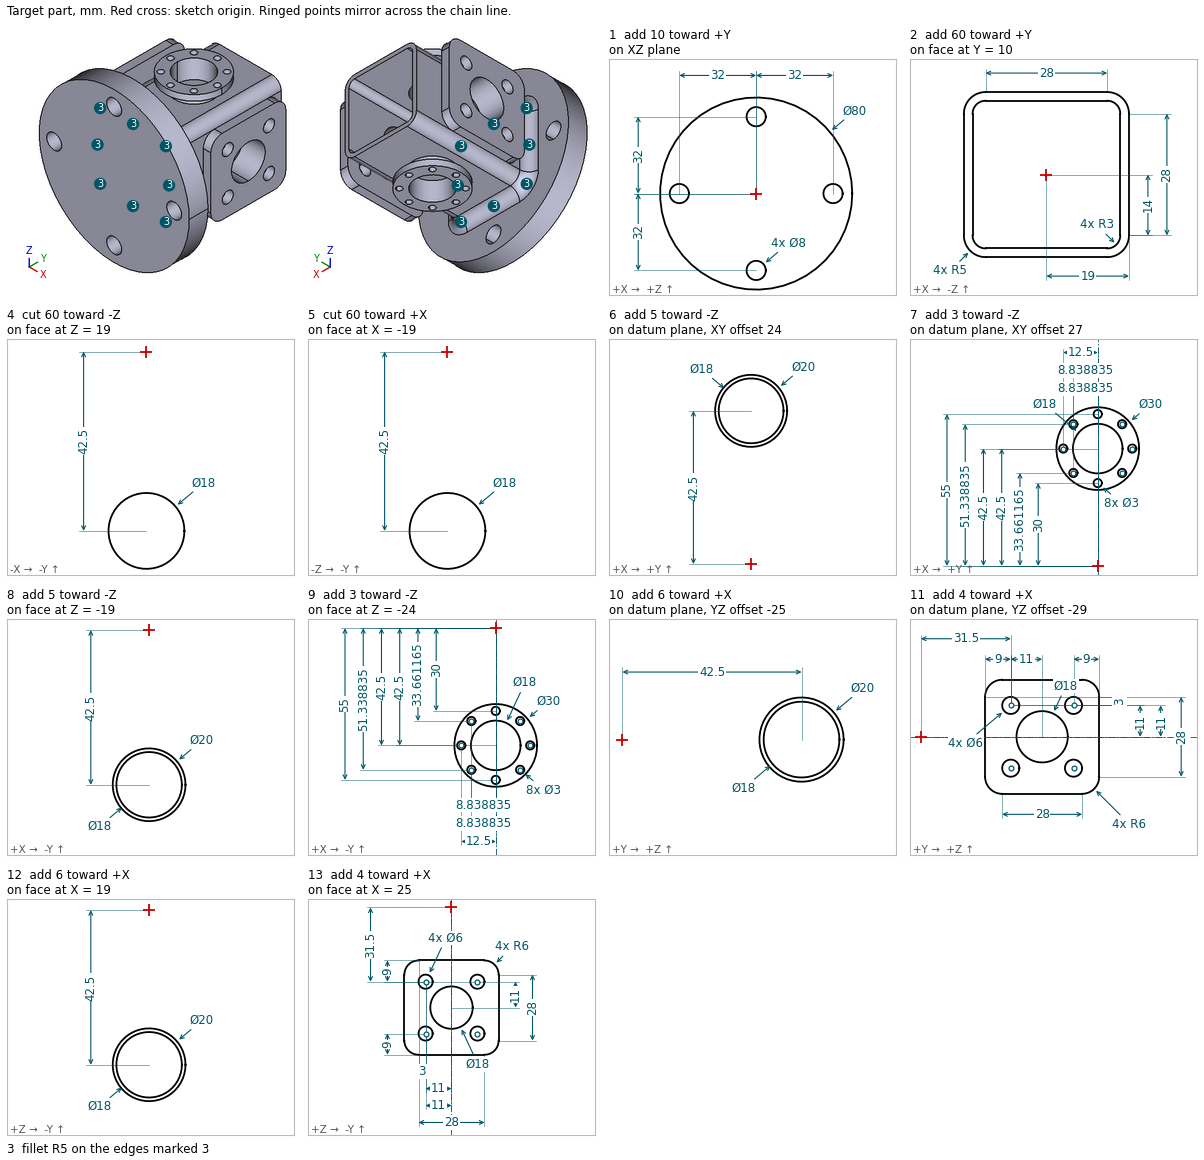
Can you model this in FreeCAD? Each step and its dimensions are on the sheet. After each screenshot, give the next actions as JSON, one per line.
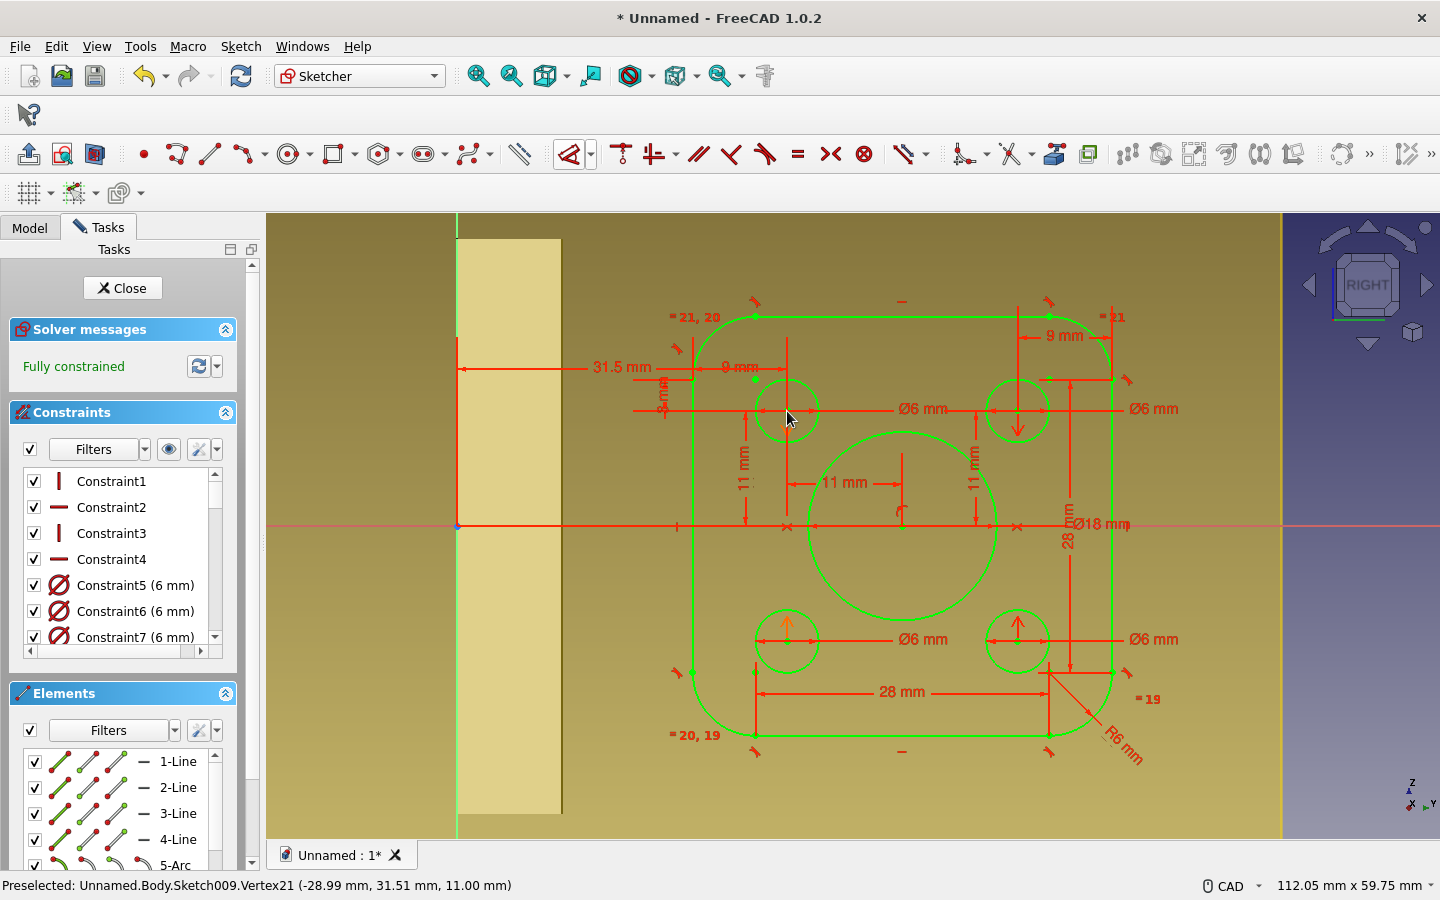
{"action": "left_click", "coordinate": [123, 288]}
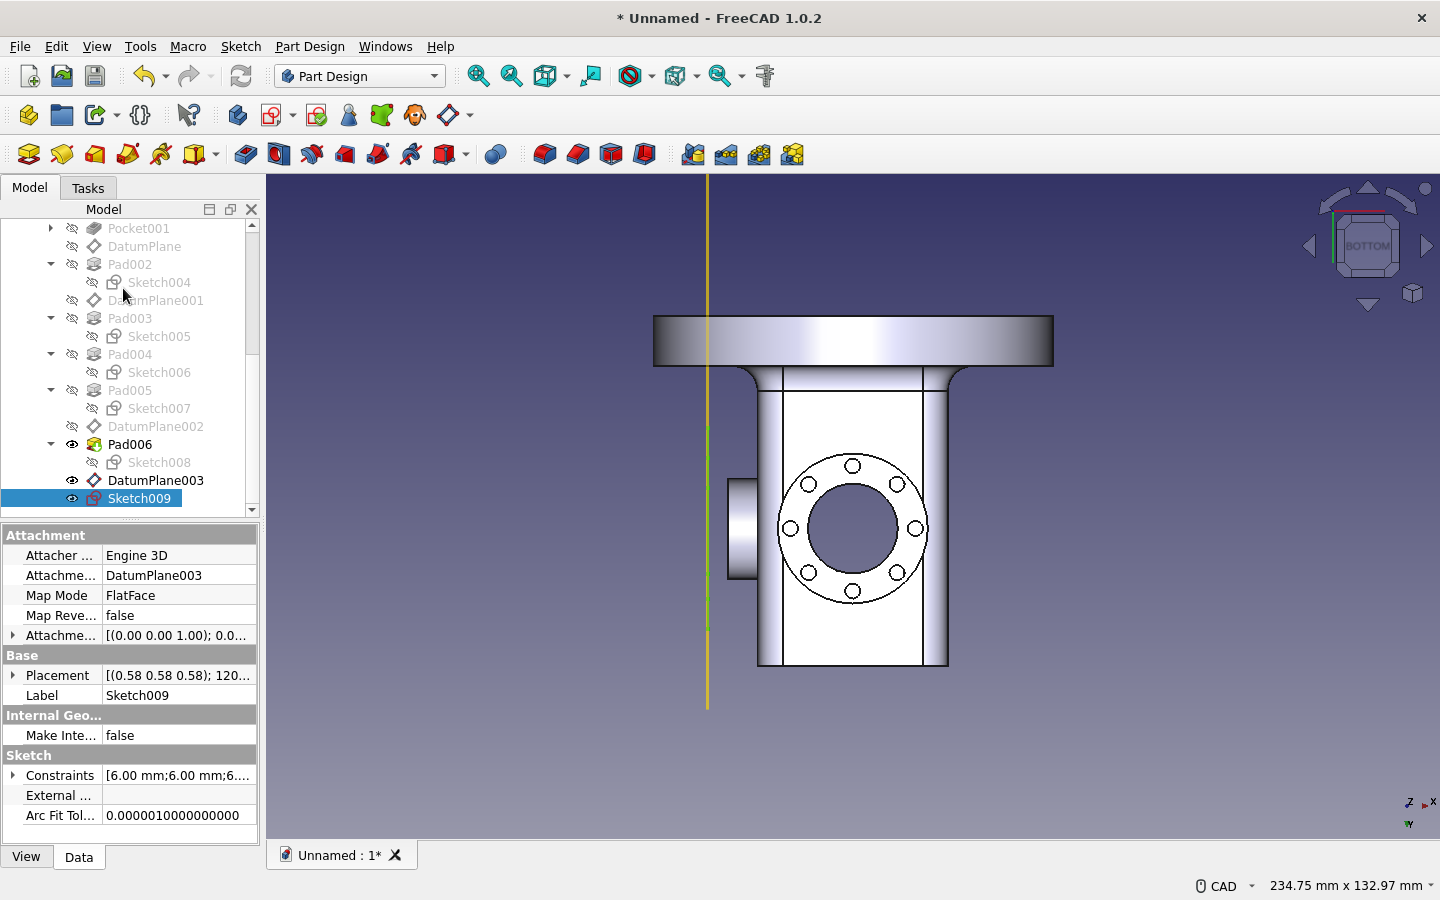
{"action": "left_click", "coordinate": [29, 154]}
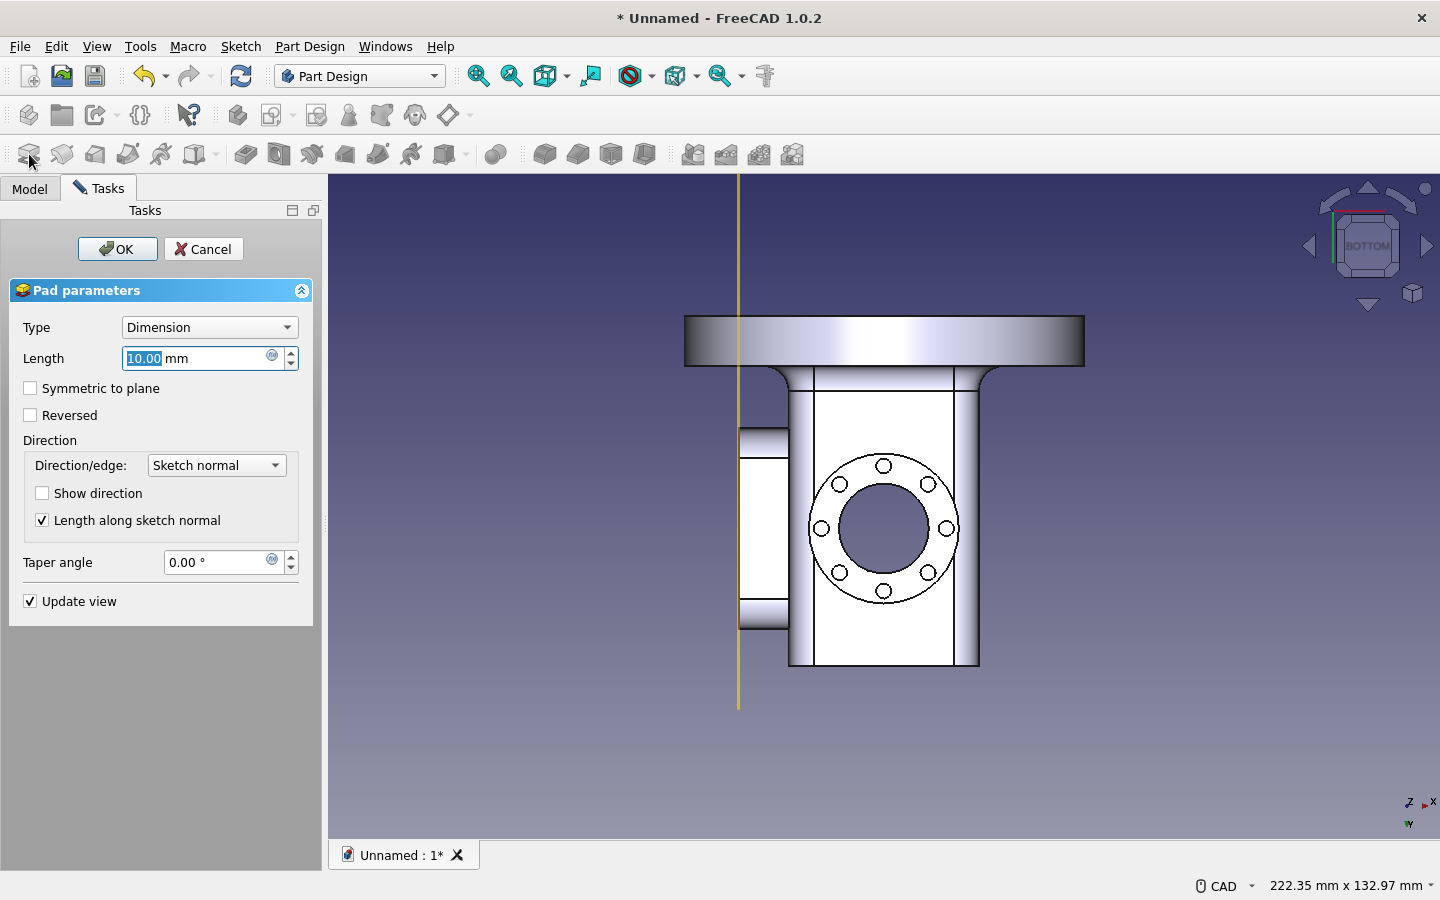
{"action": "type", "text": "4"}
{"action": "key", "text": "Tab"}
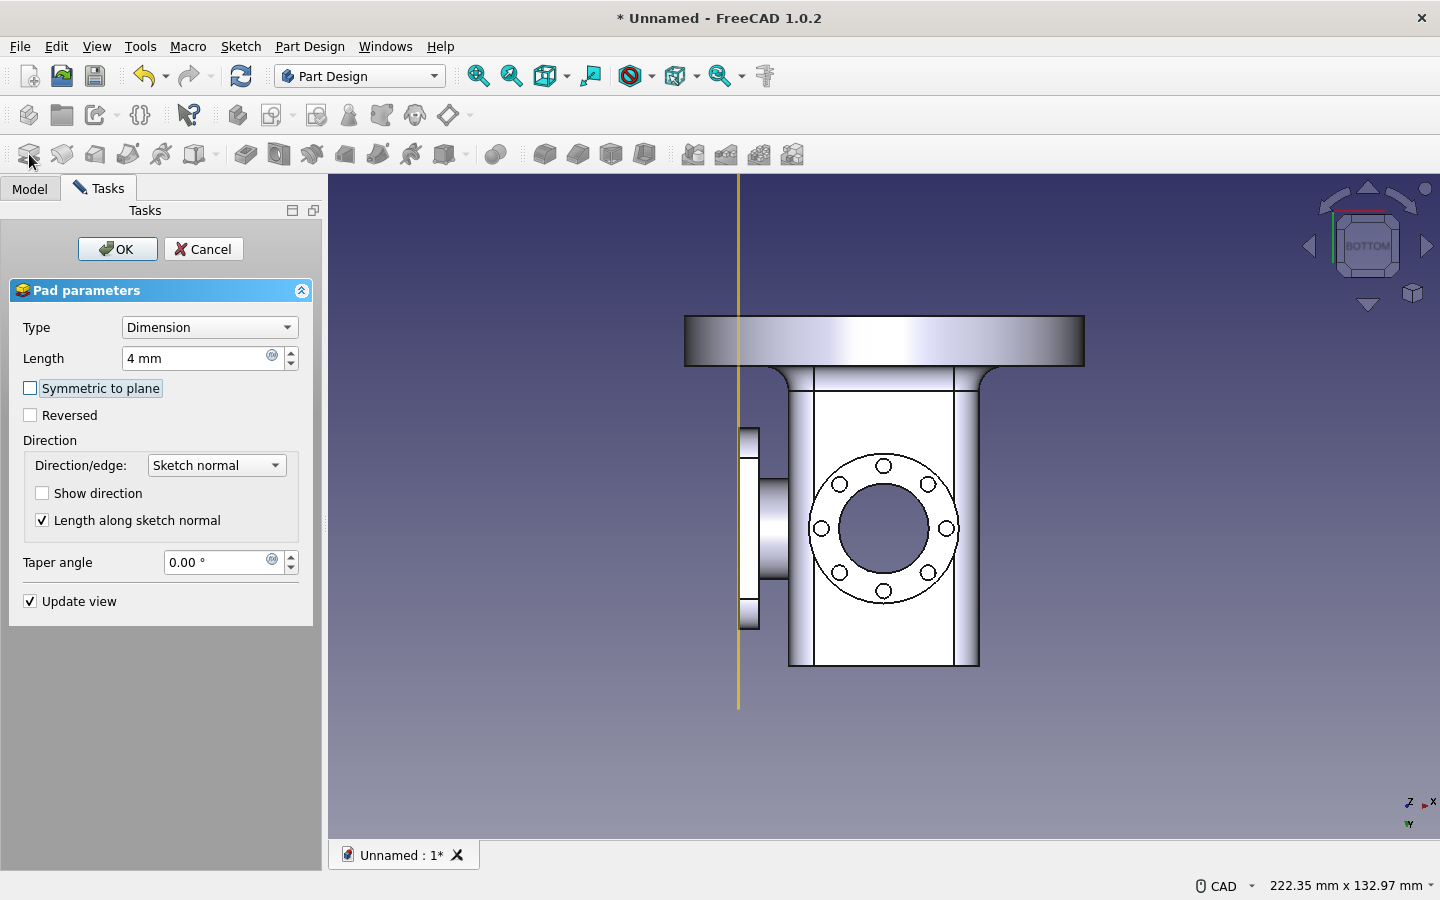
{"action": "left_click", "coordinate": [118, 249]}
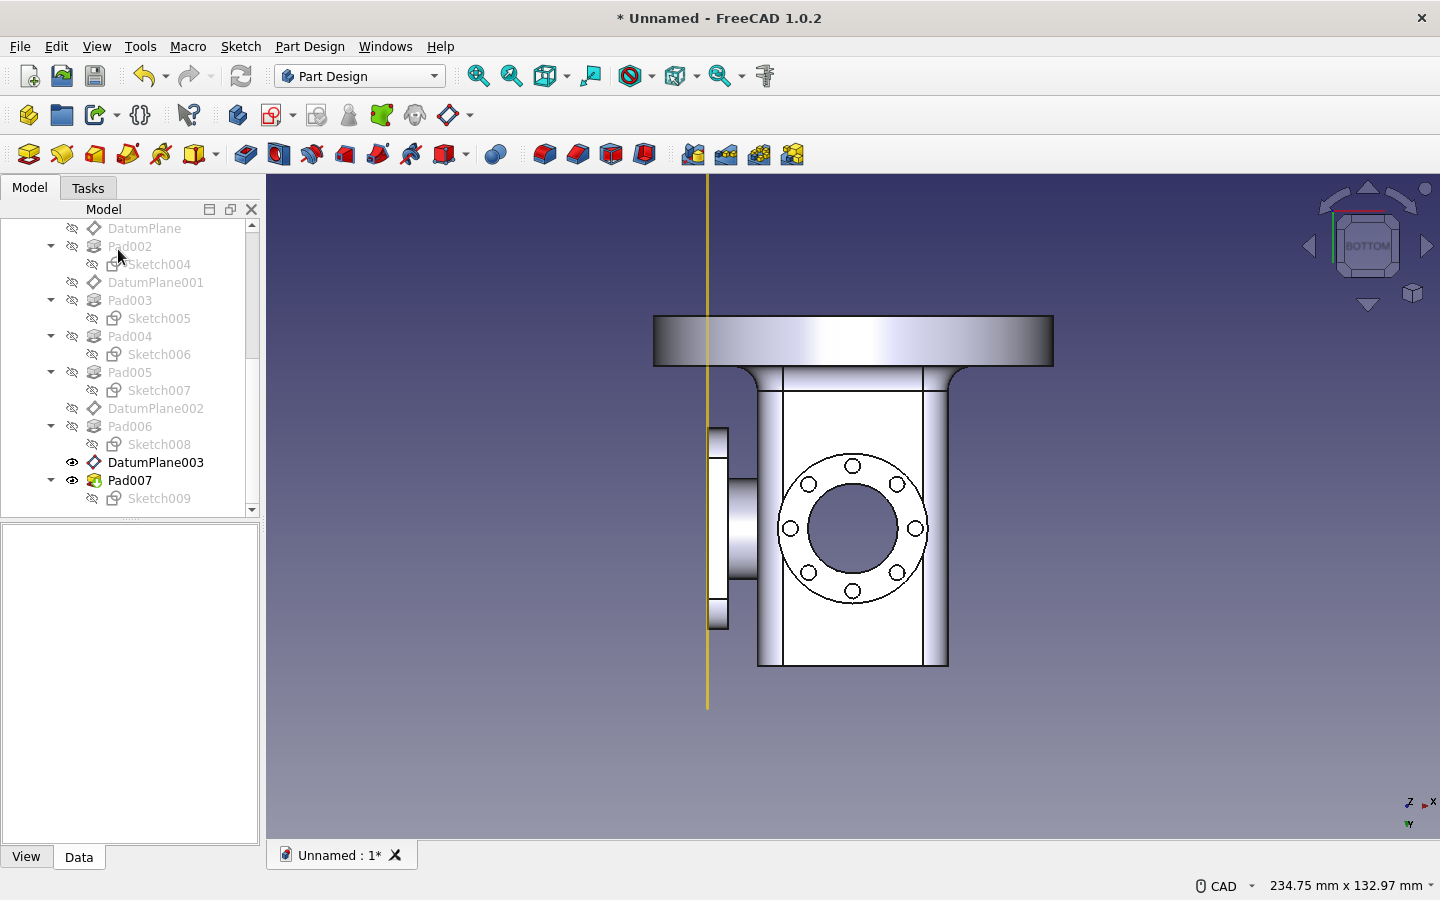
{"action": "left_click", "coordinate": [117, 462]}
{"action": "key", "text": "space"}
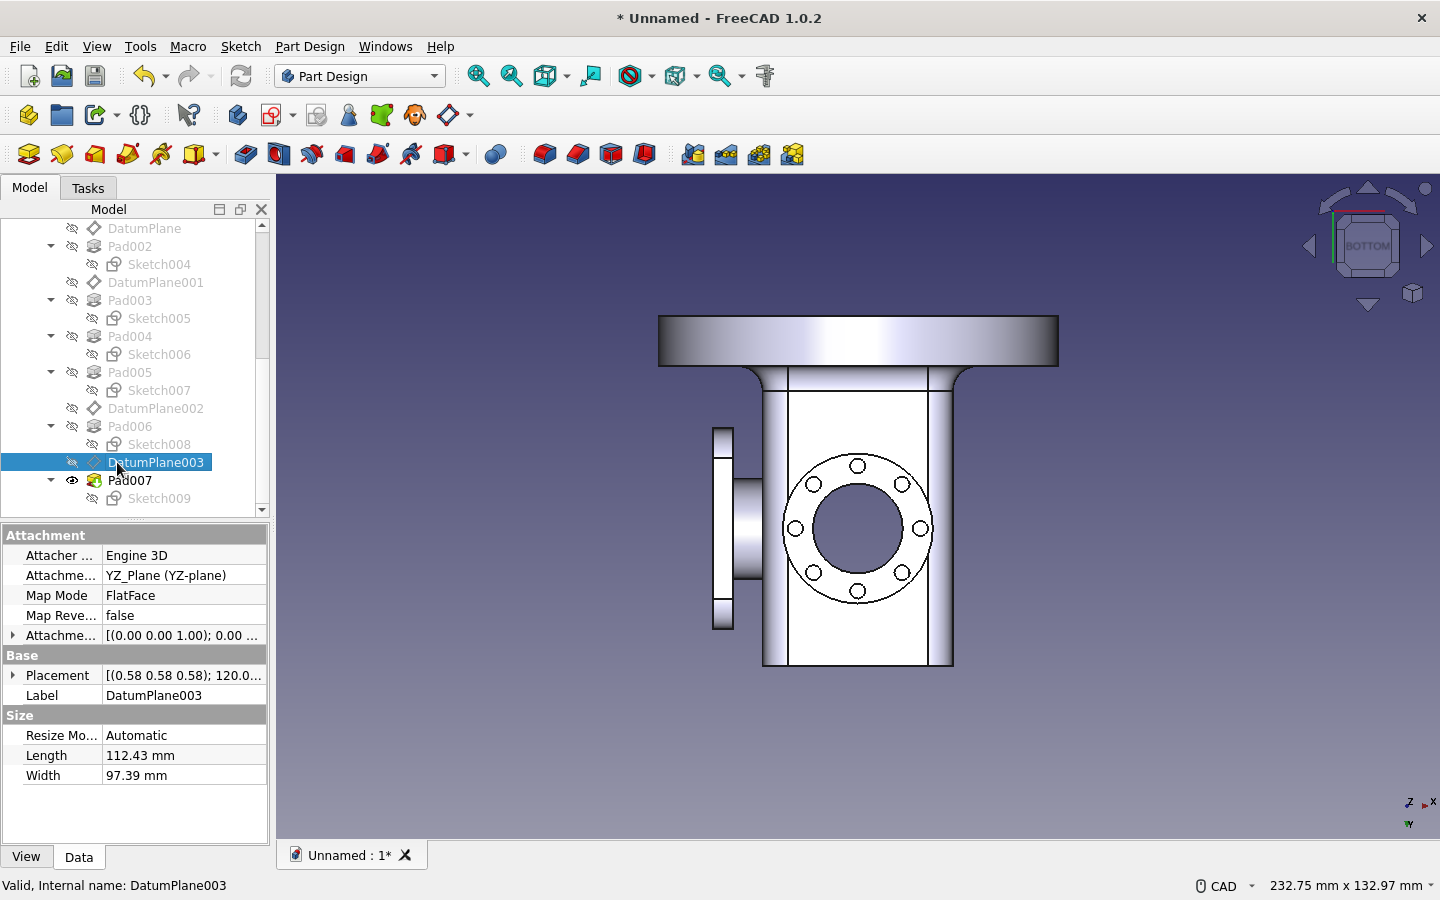
{"action": "key", "text": "0"}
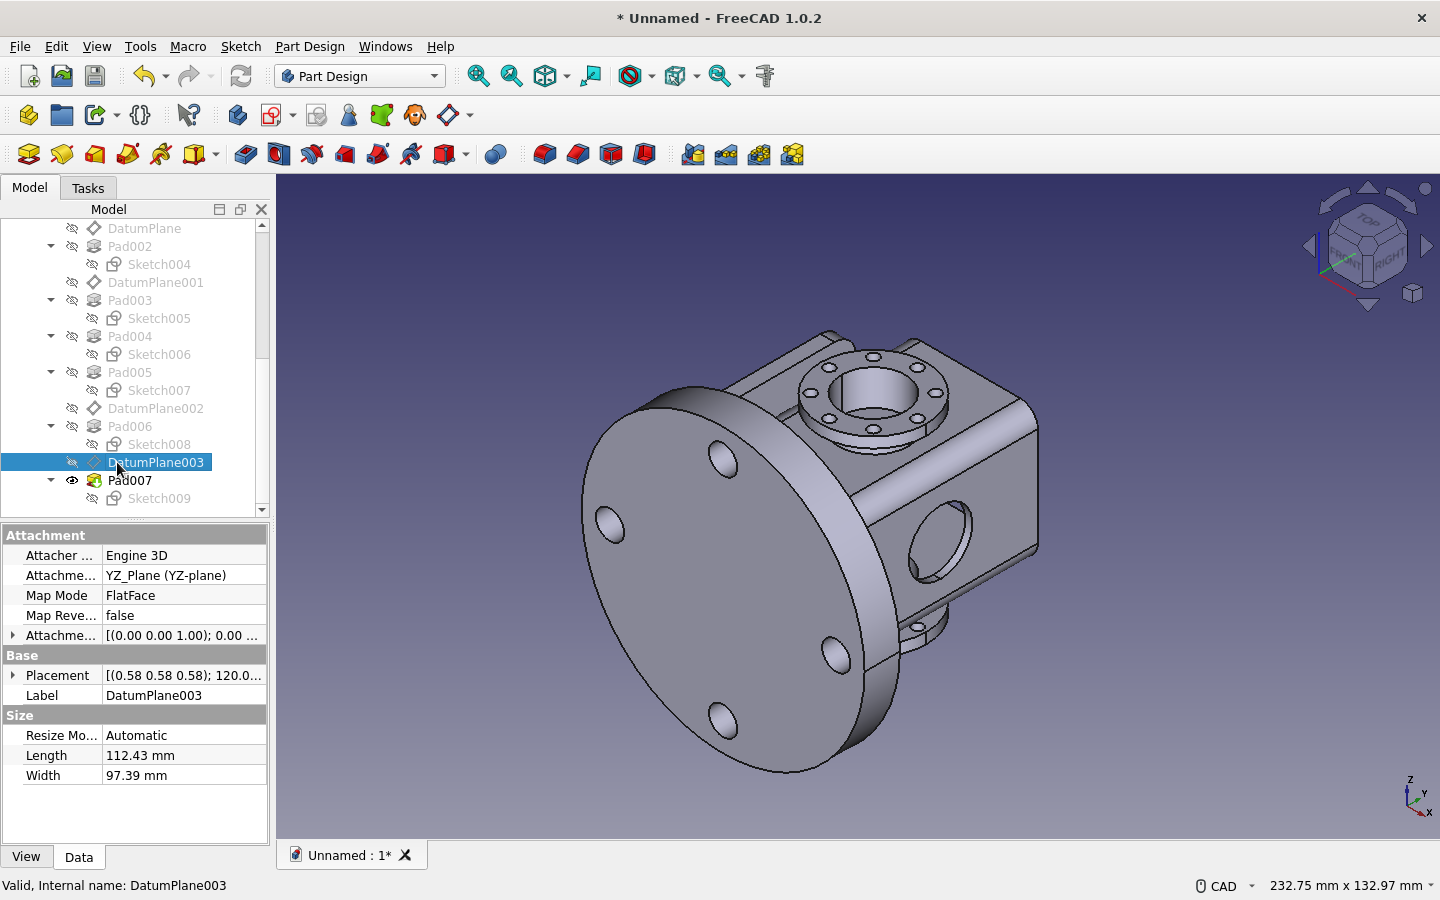
{"action": "left_click", "coordinate": [996, 493]}